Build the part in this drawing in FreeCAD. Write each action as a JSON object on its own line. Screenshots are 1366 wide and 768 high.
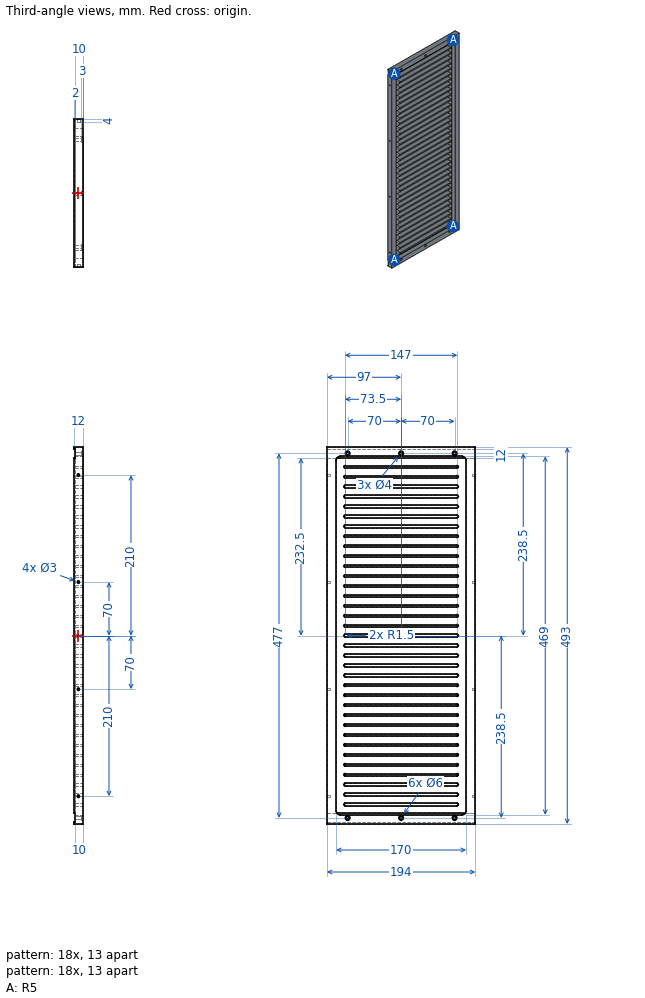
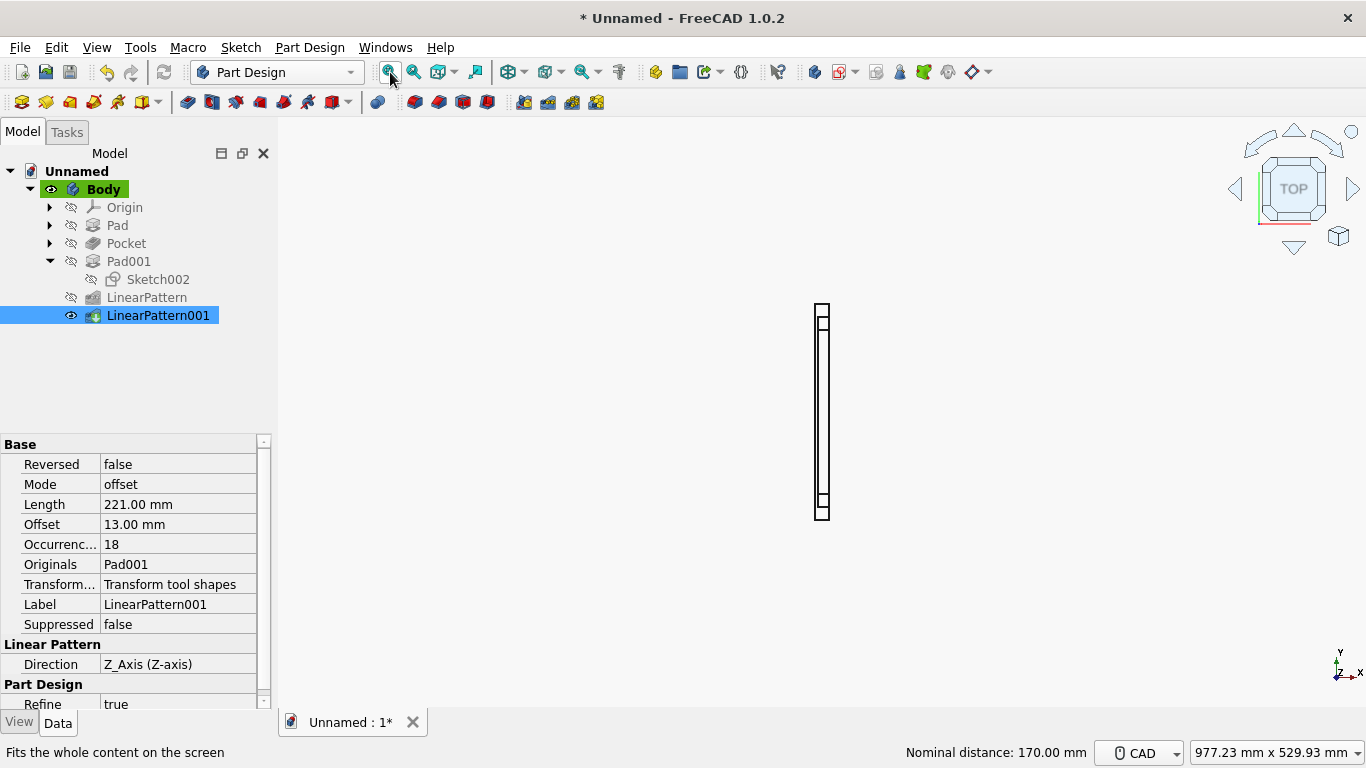
{"action": "left_click", "coordinate": [822, 506], "text": "ctrl"}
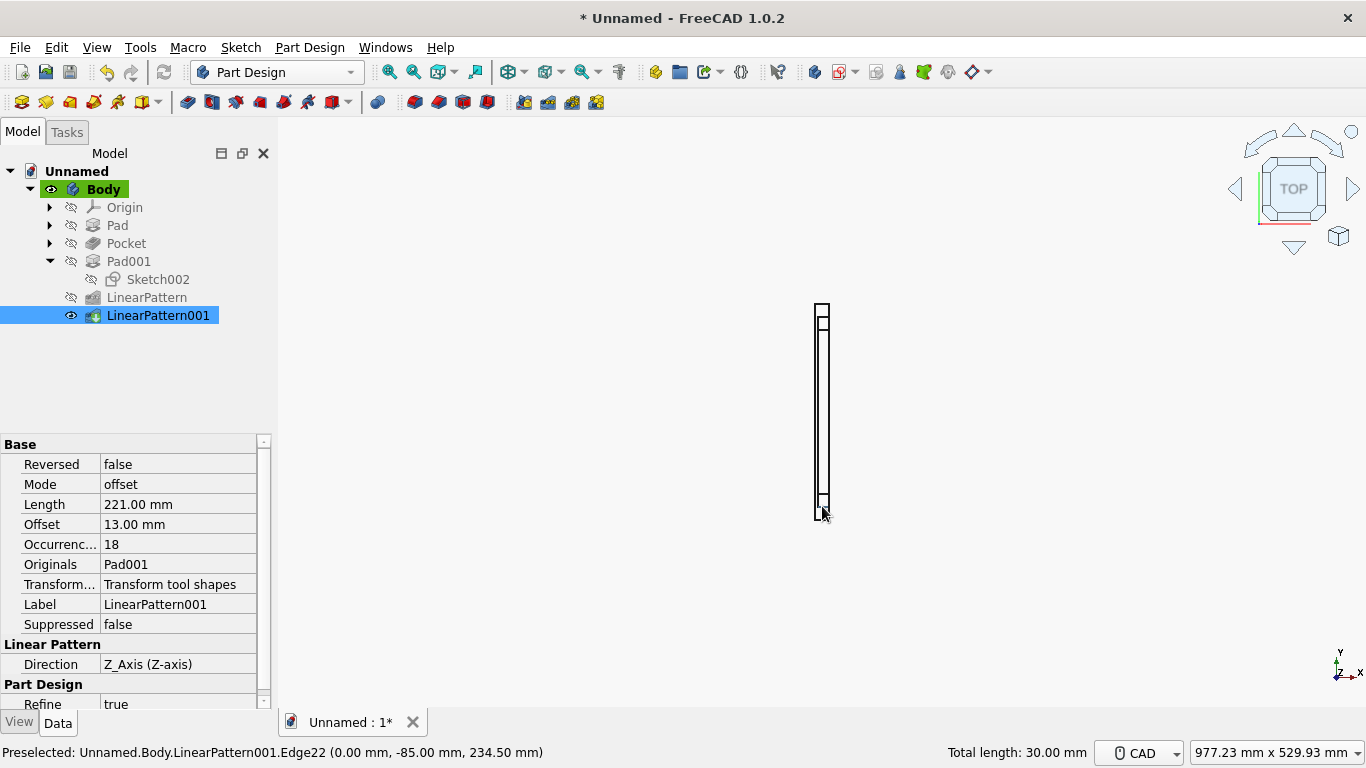
{"action": "left_click", "coordinate": [822, 316], "text": "ctrl"}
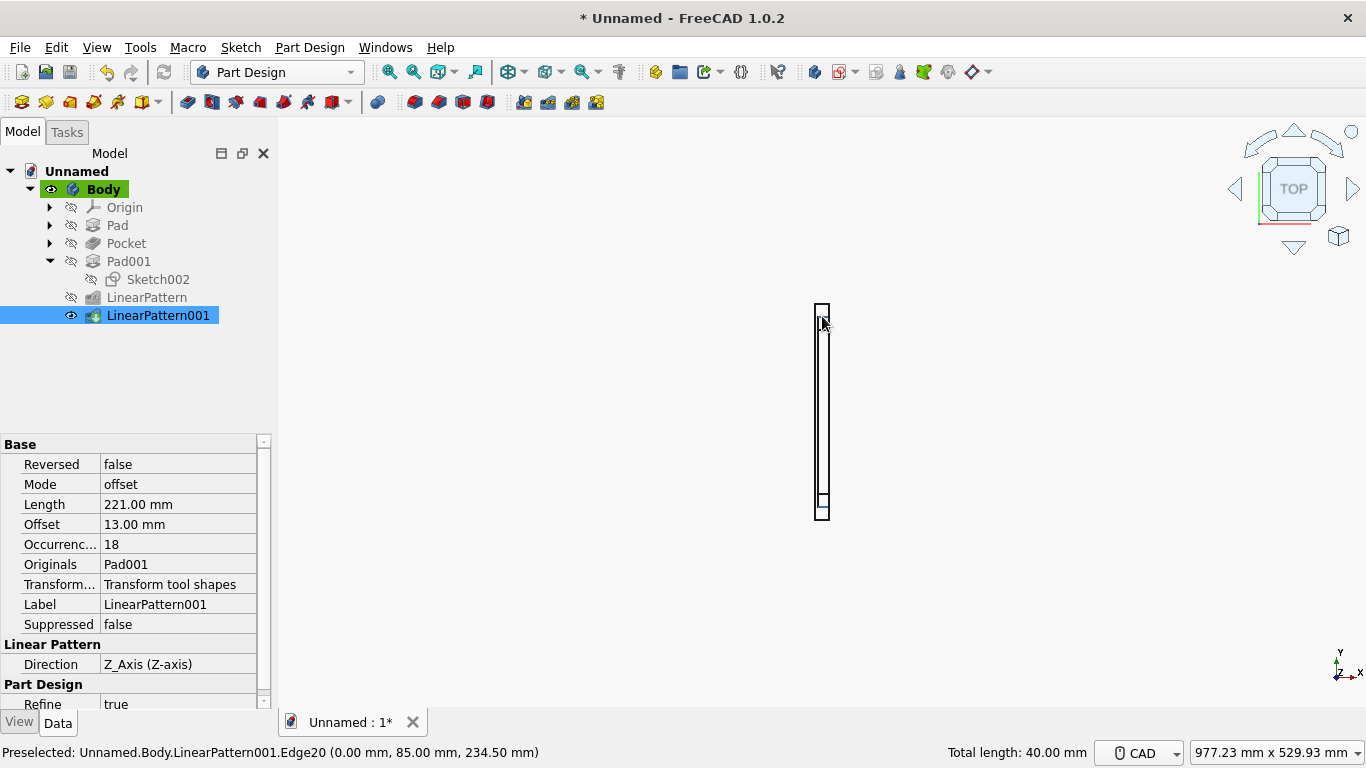
{"action": "key", "text": "v 1"}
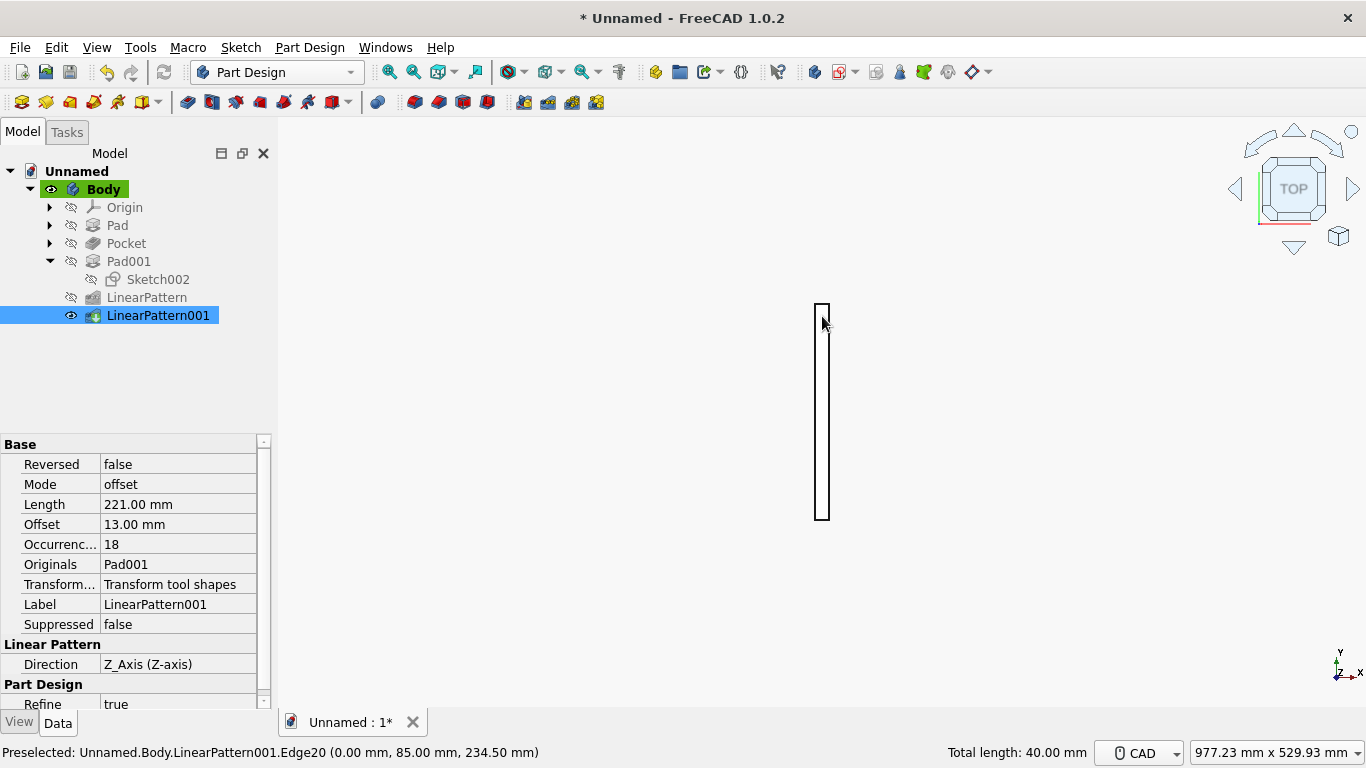
{"action": "left_click", "coordinate": [416, 102]}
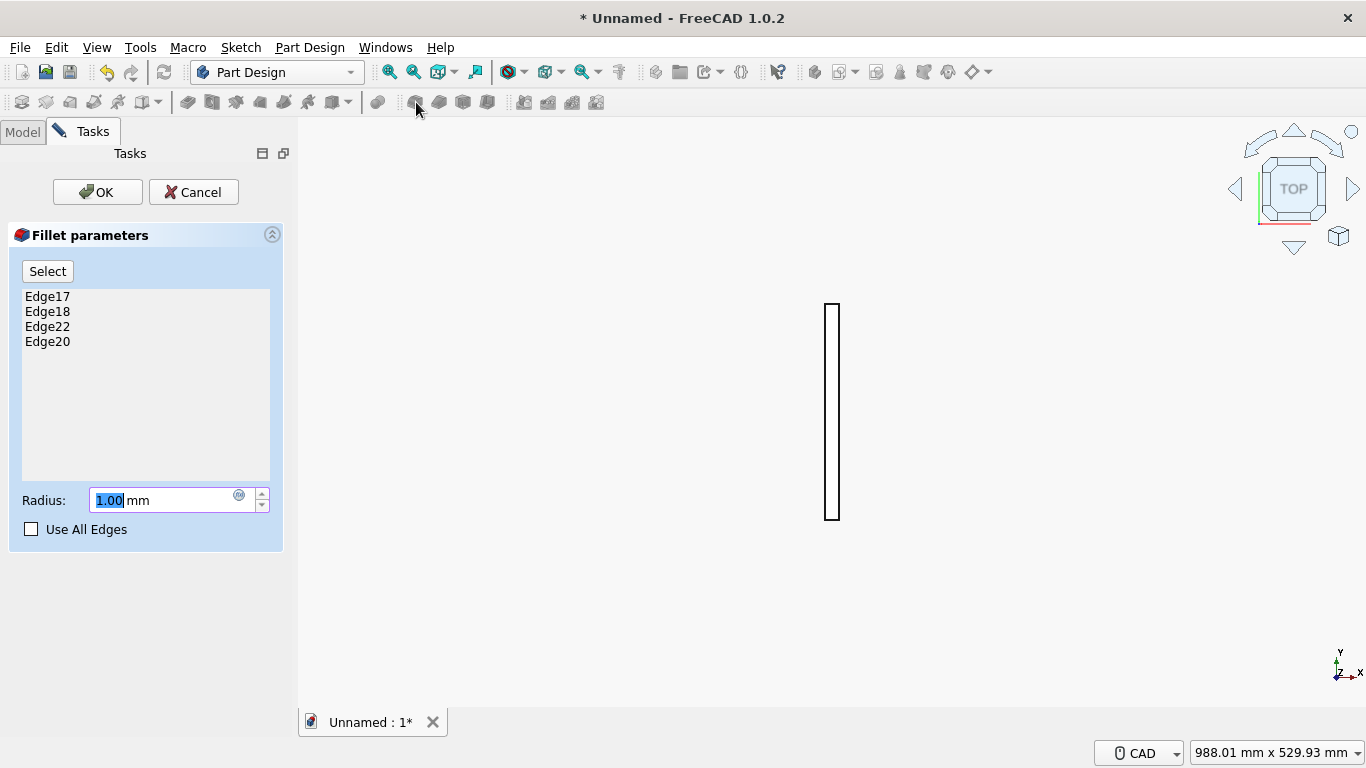
{"action": "type", "text": "5"}
{"action": "key", "text": "Tab"}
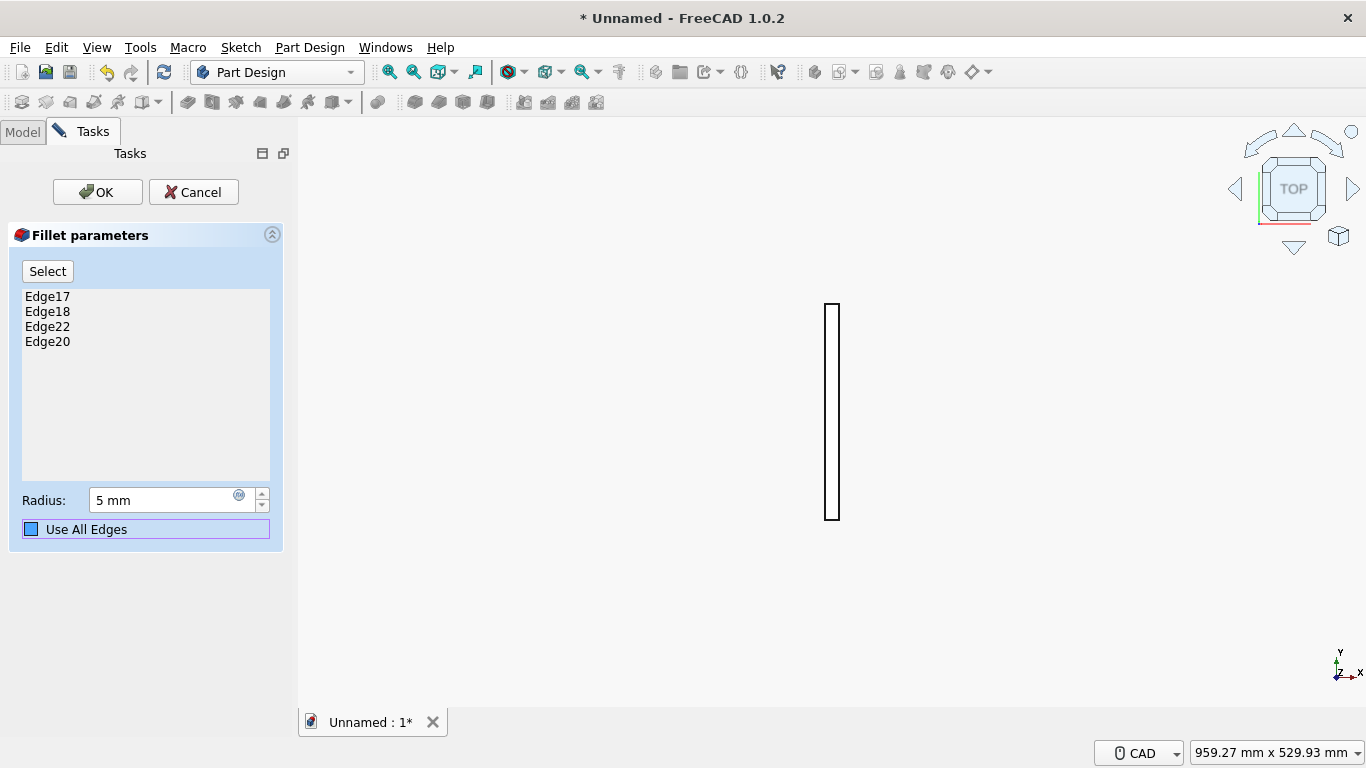
{"action": "left_click", "coordinate": [98, 192]}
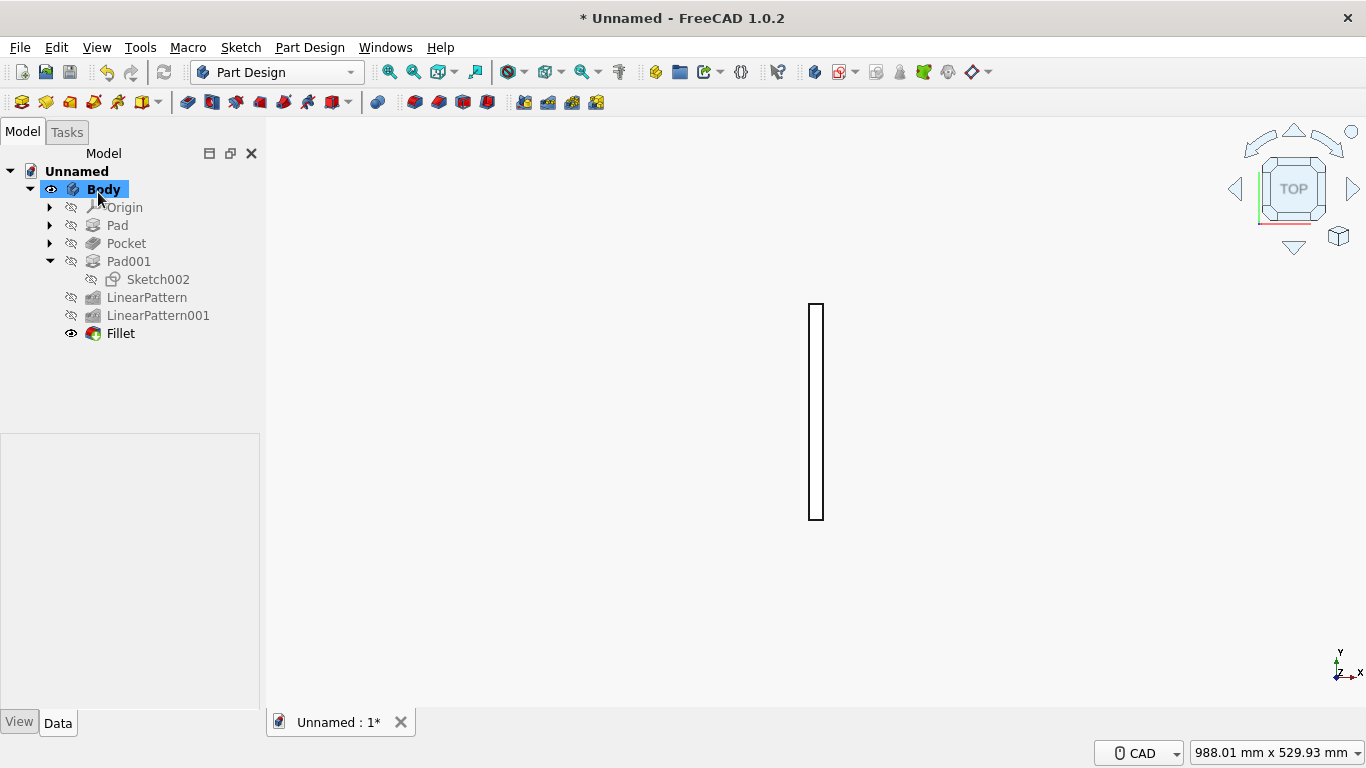
{"action": "left_click", "coordinate": [390, 72]}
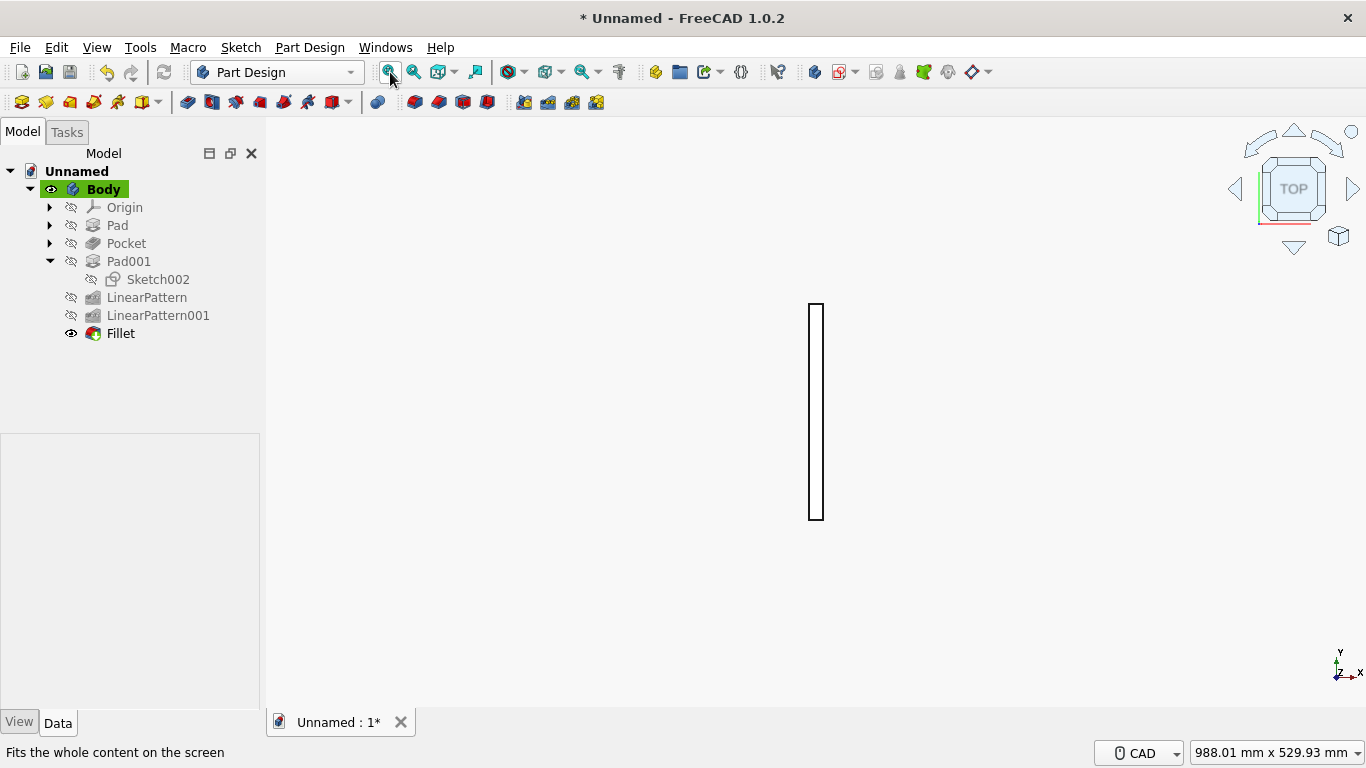
{"action": "key", "text": "0"}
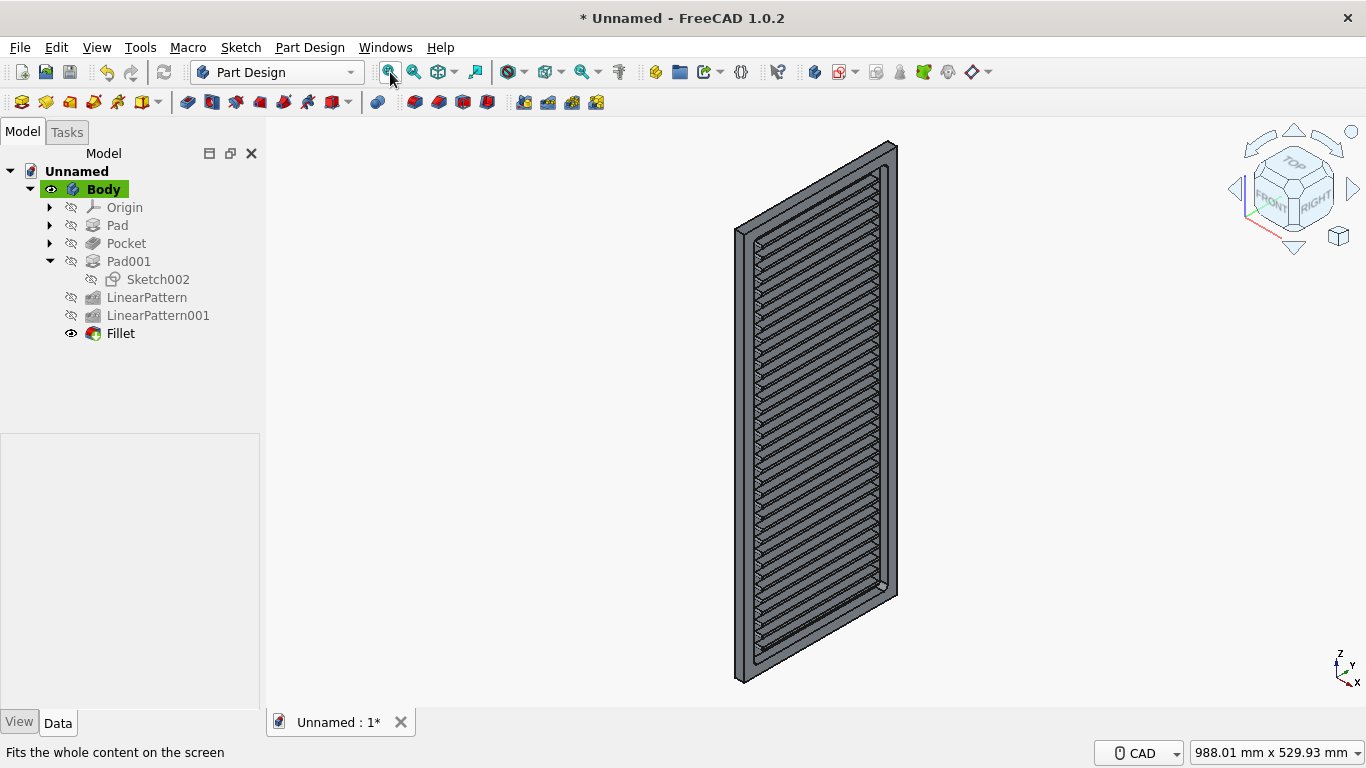
{"action": "key", "text": "3"}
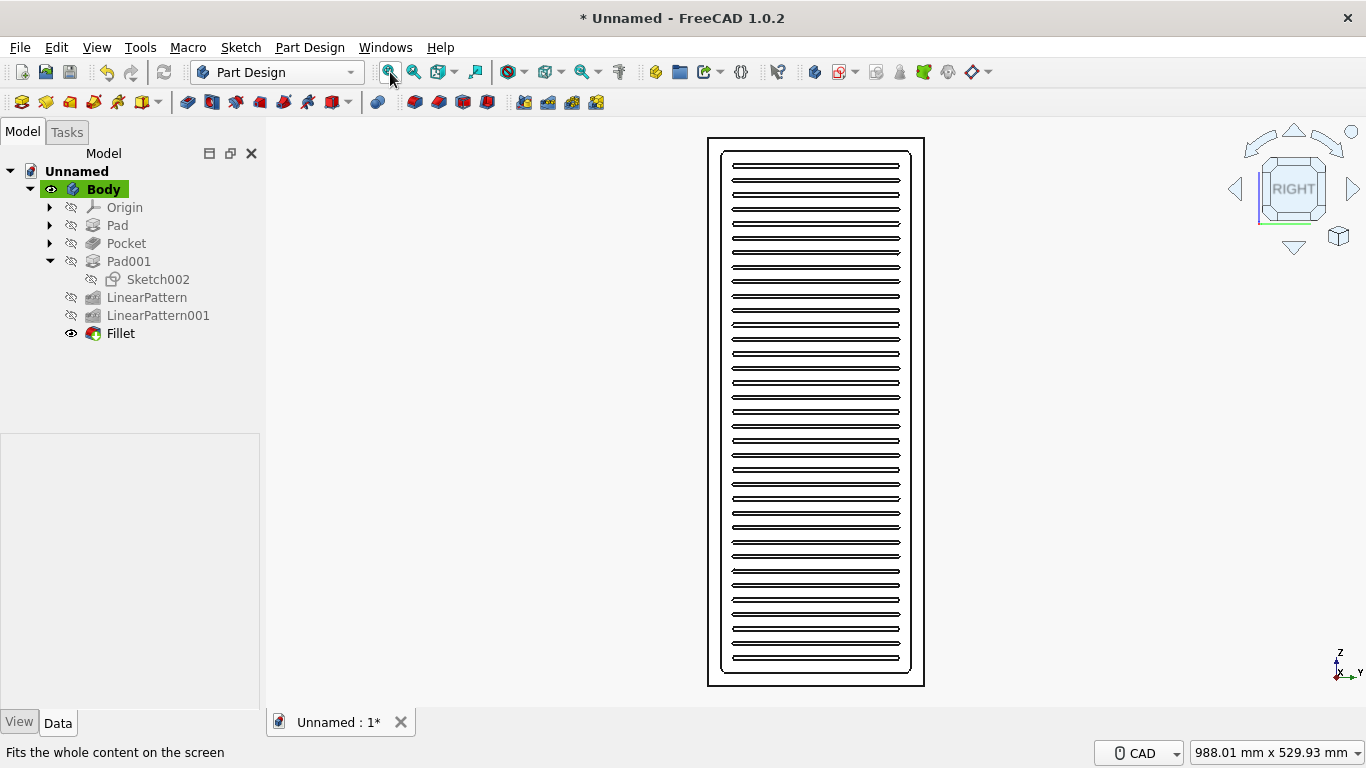
{"action": "key", "text": "2"}